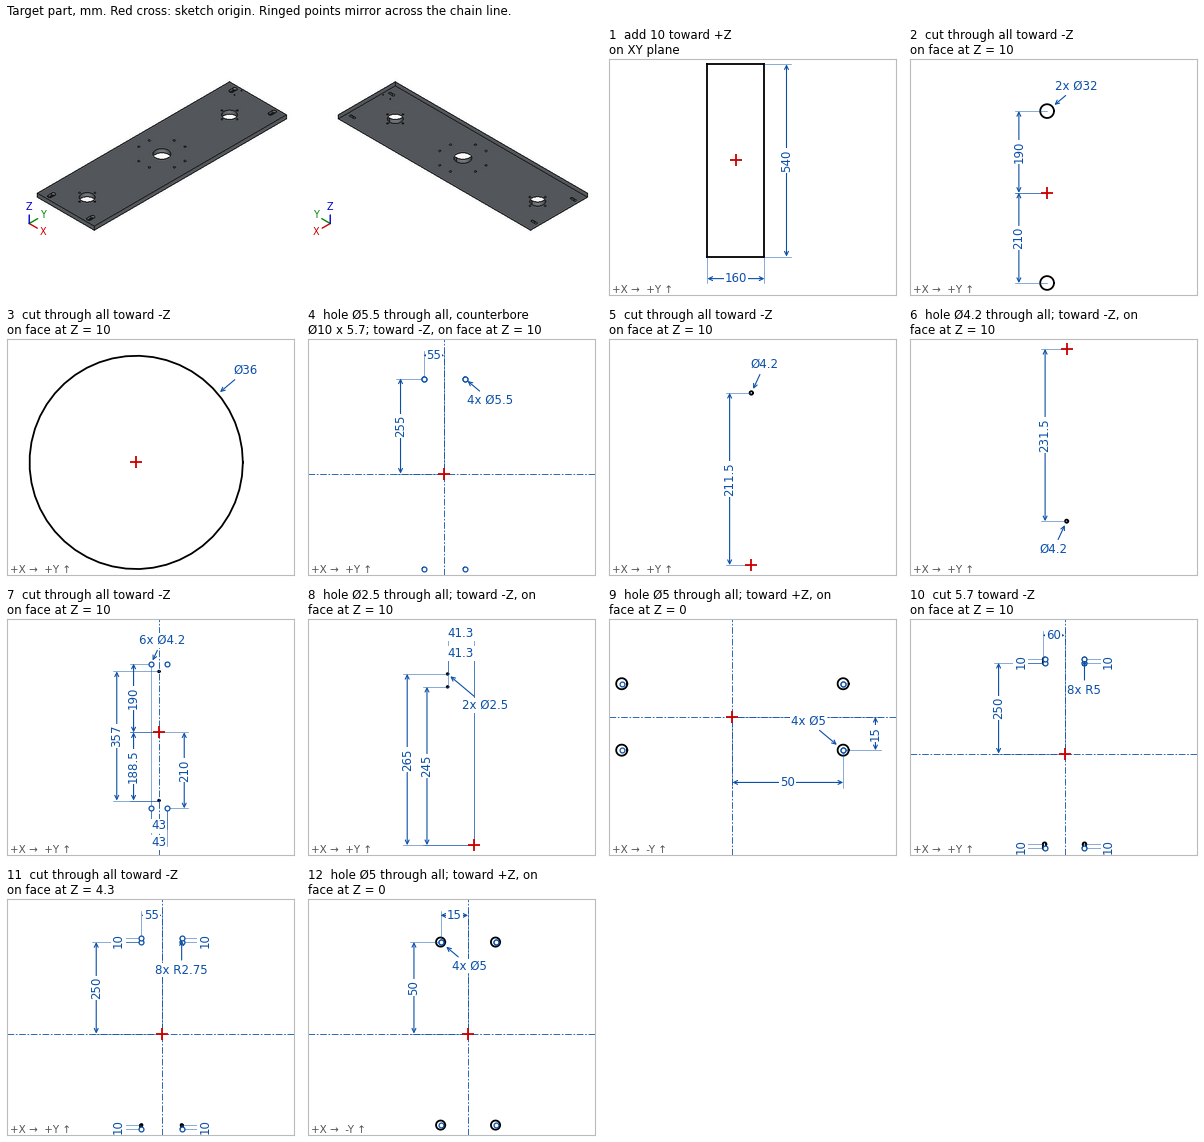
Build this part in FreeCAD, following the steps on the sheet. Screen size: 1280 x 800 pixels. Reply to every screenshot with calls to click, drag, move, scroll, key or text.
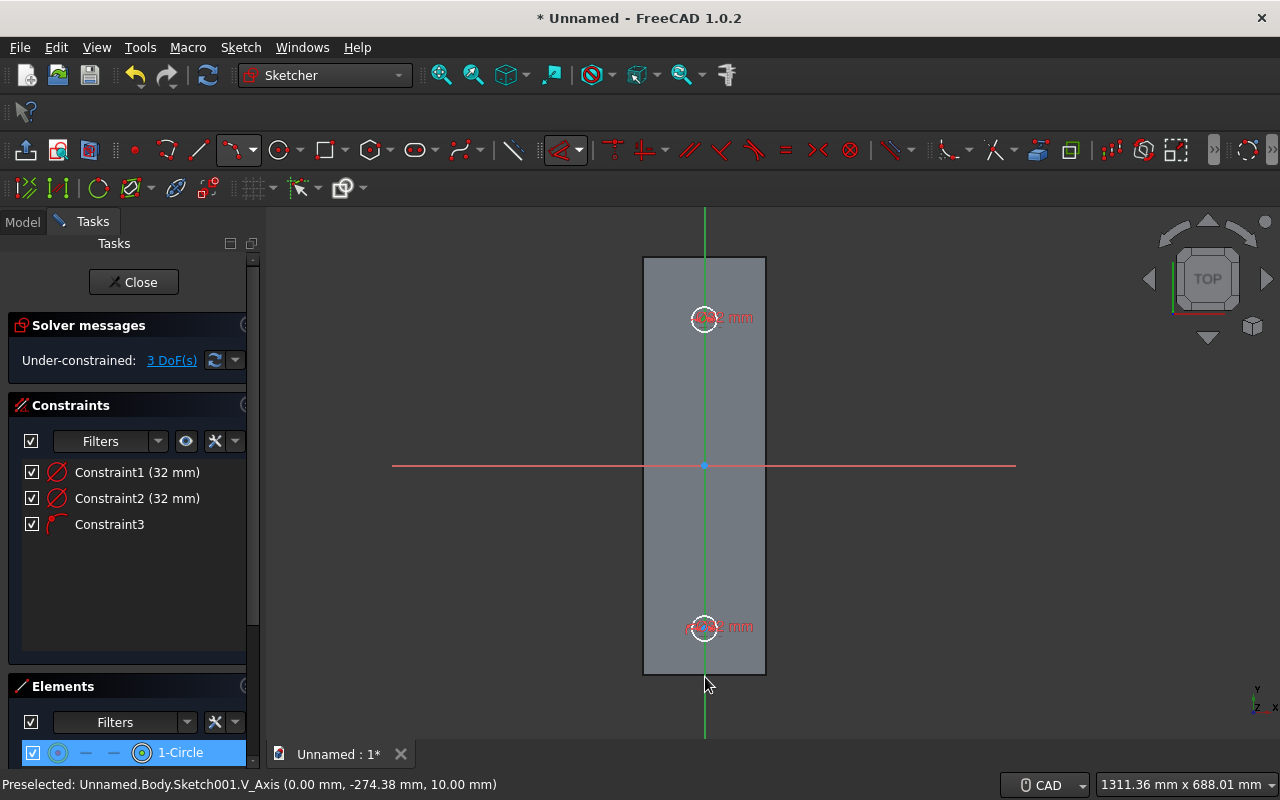
click(614, 150)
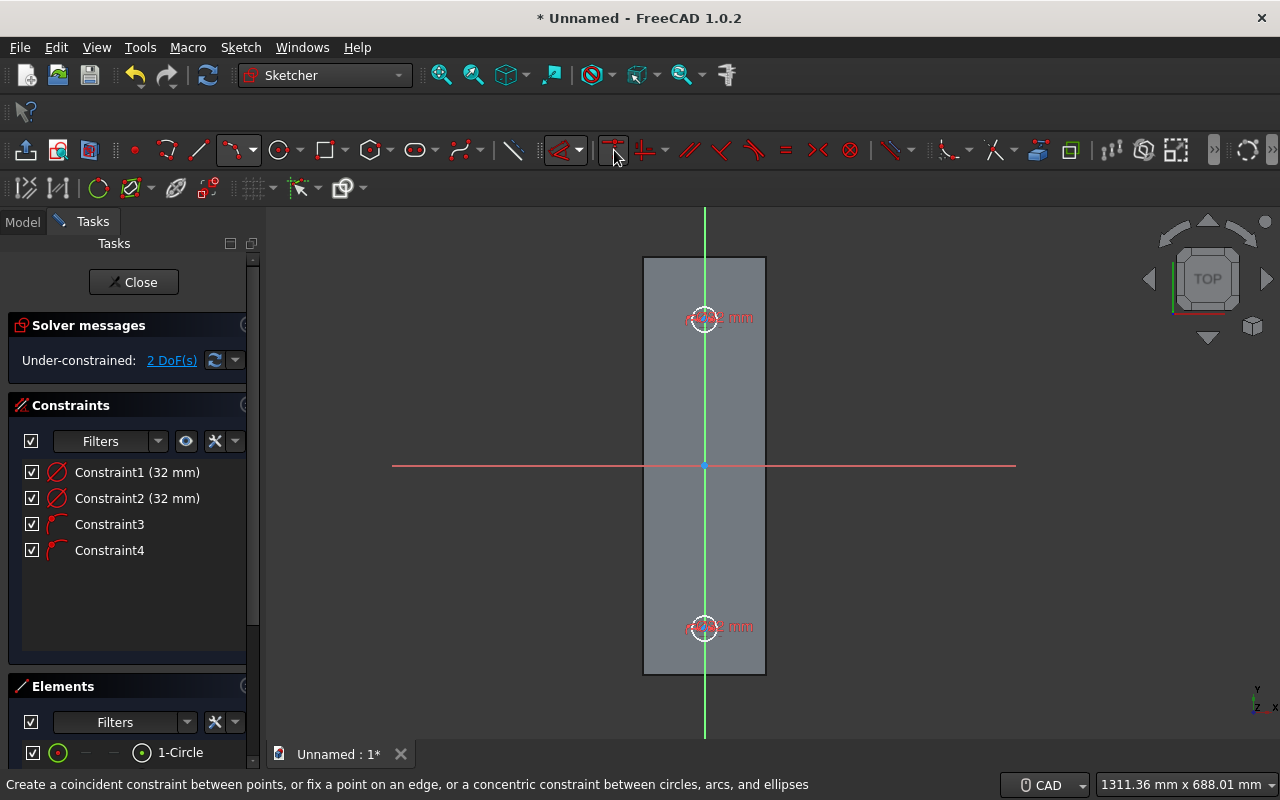
click(560, 150)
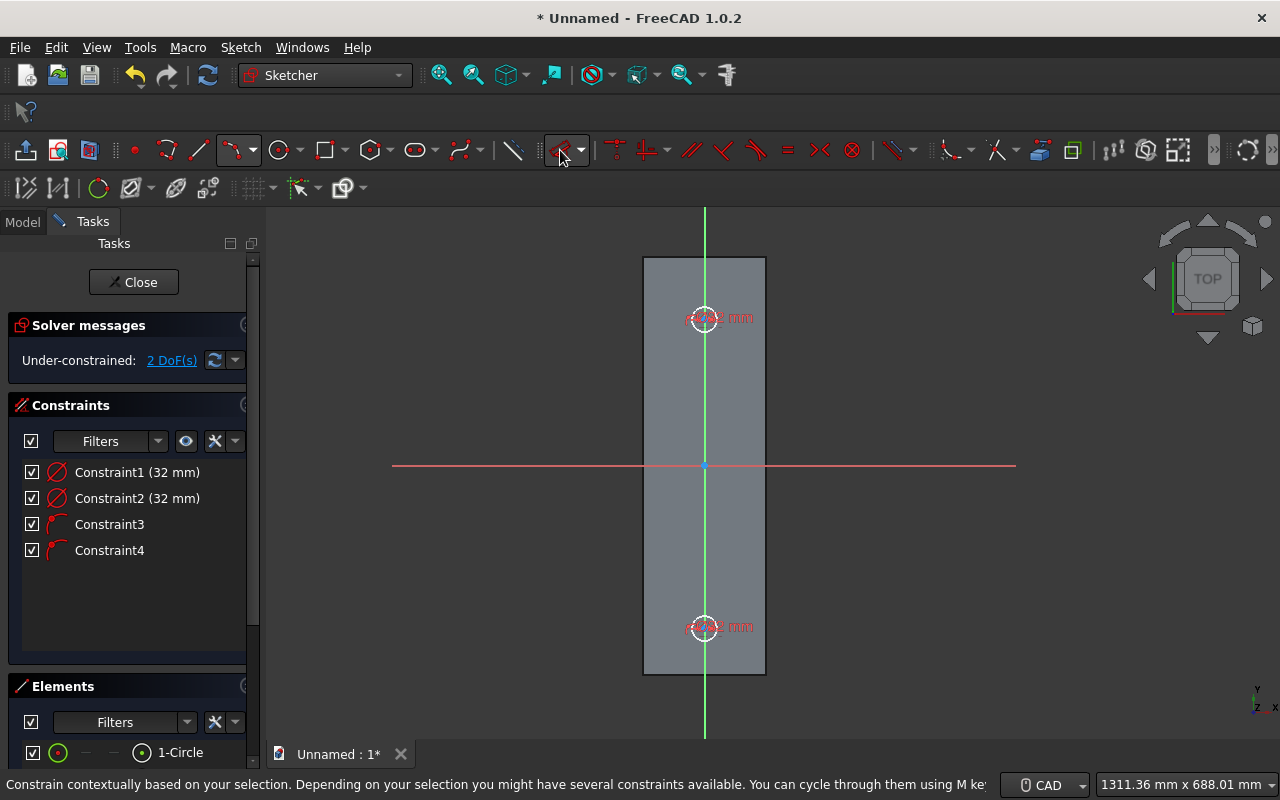
click(705, 320)
click(739, 393)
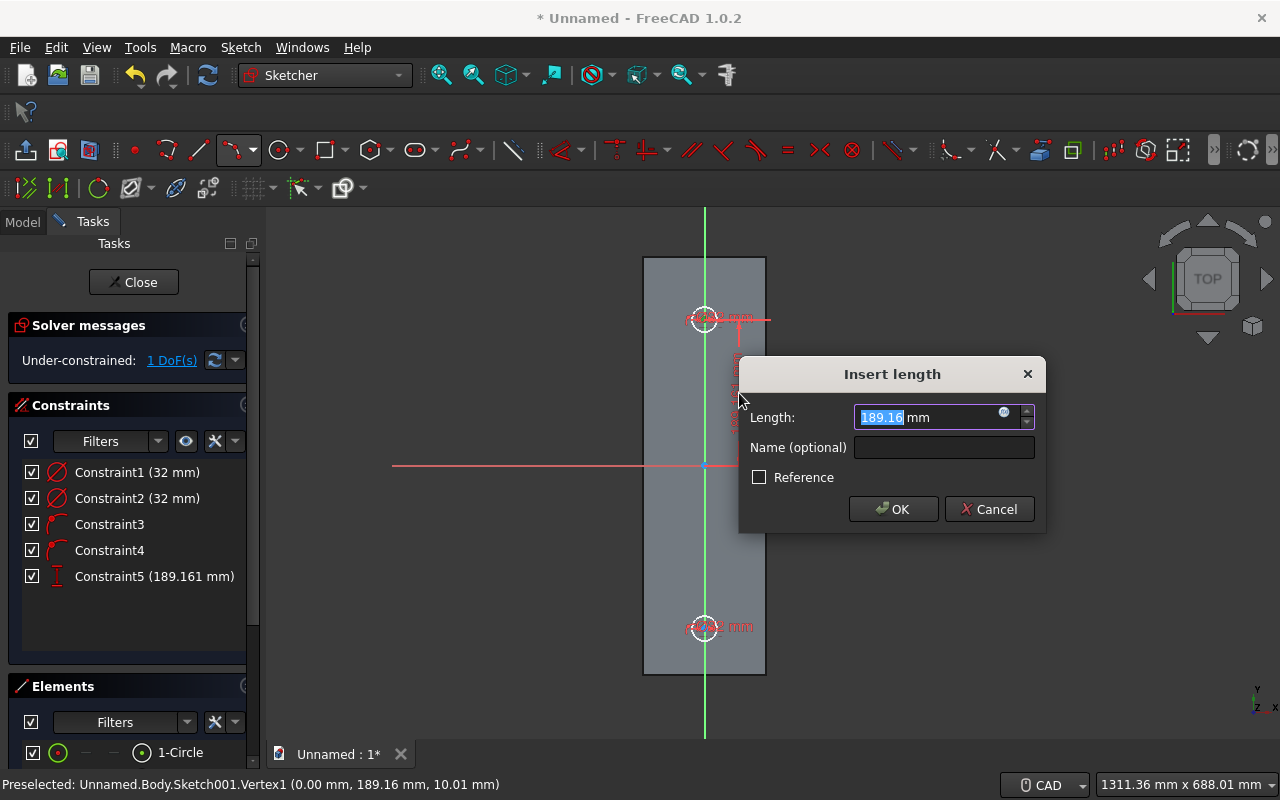
text(190)
key(Return)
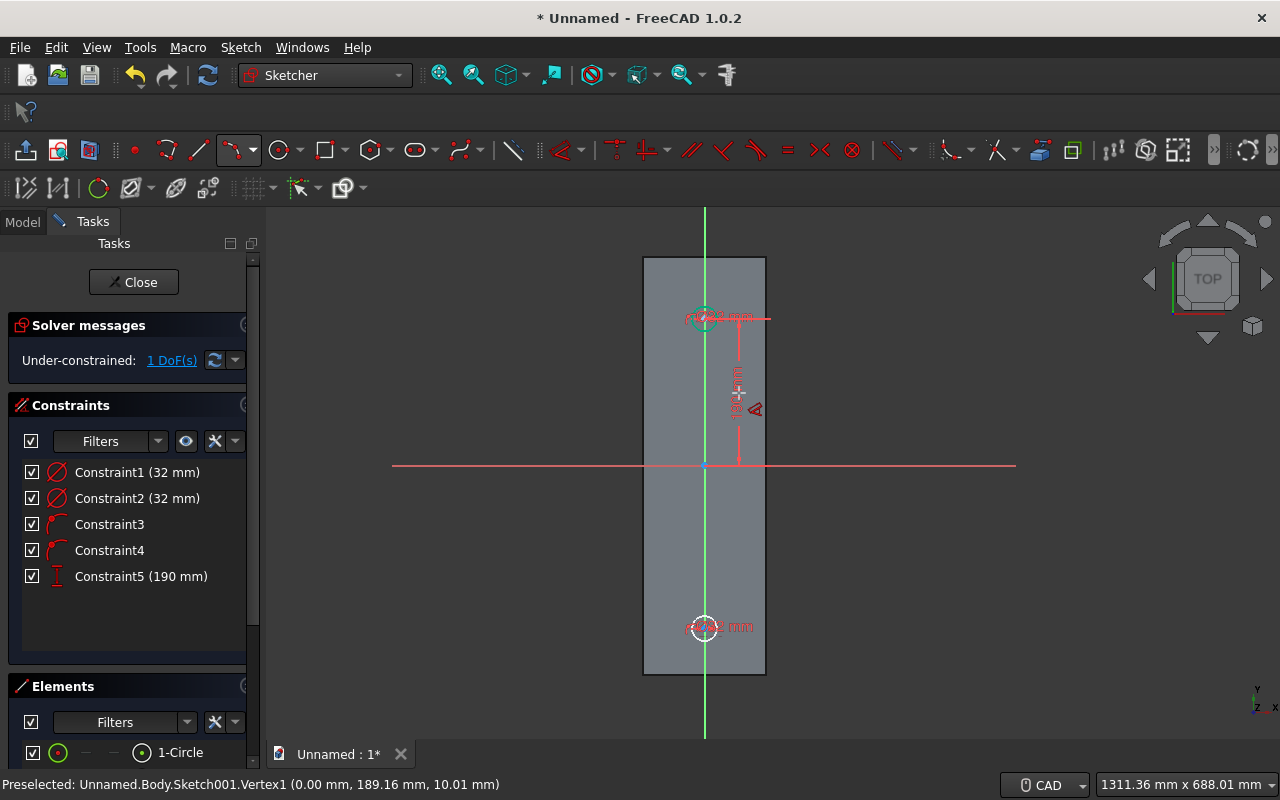
click(705, 629)
click(739, 547)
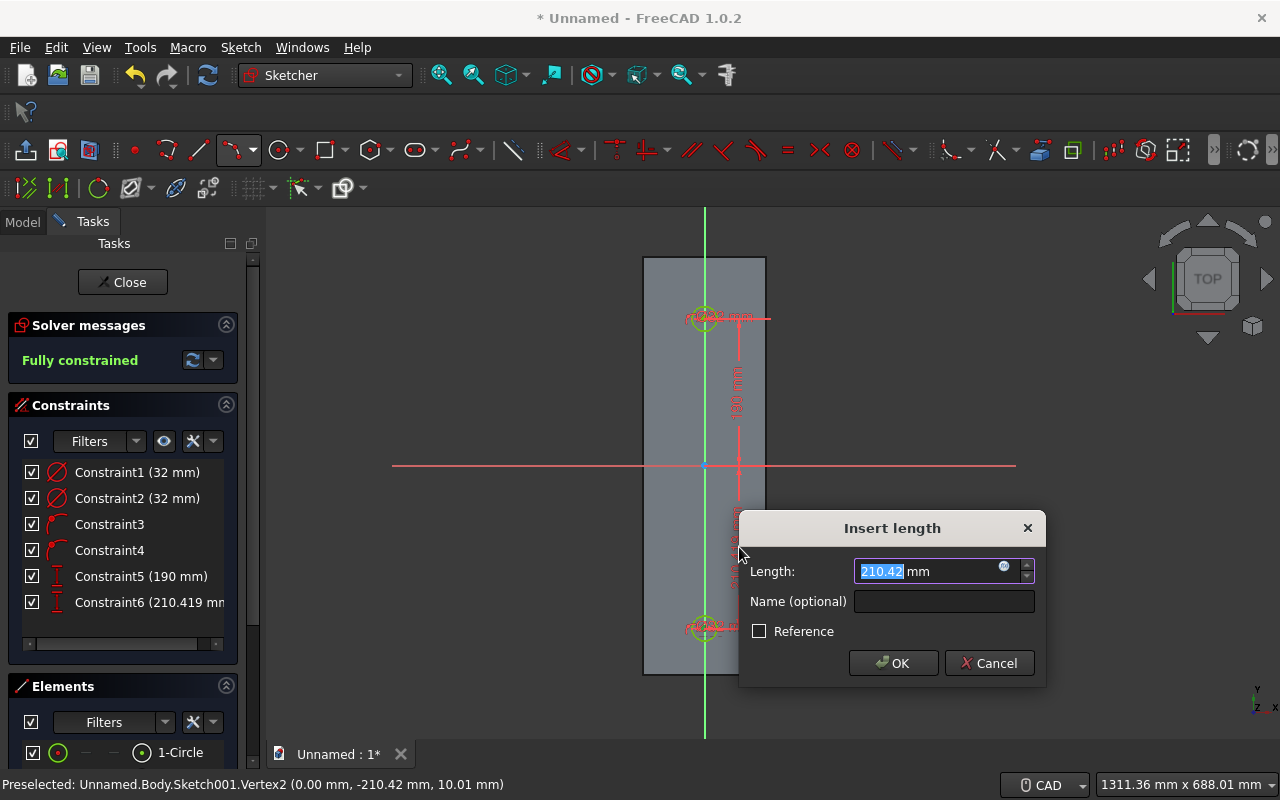
text(210)
key(Return)
key(Escape)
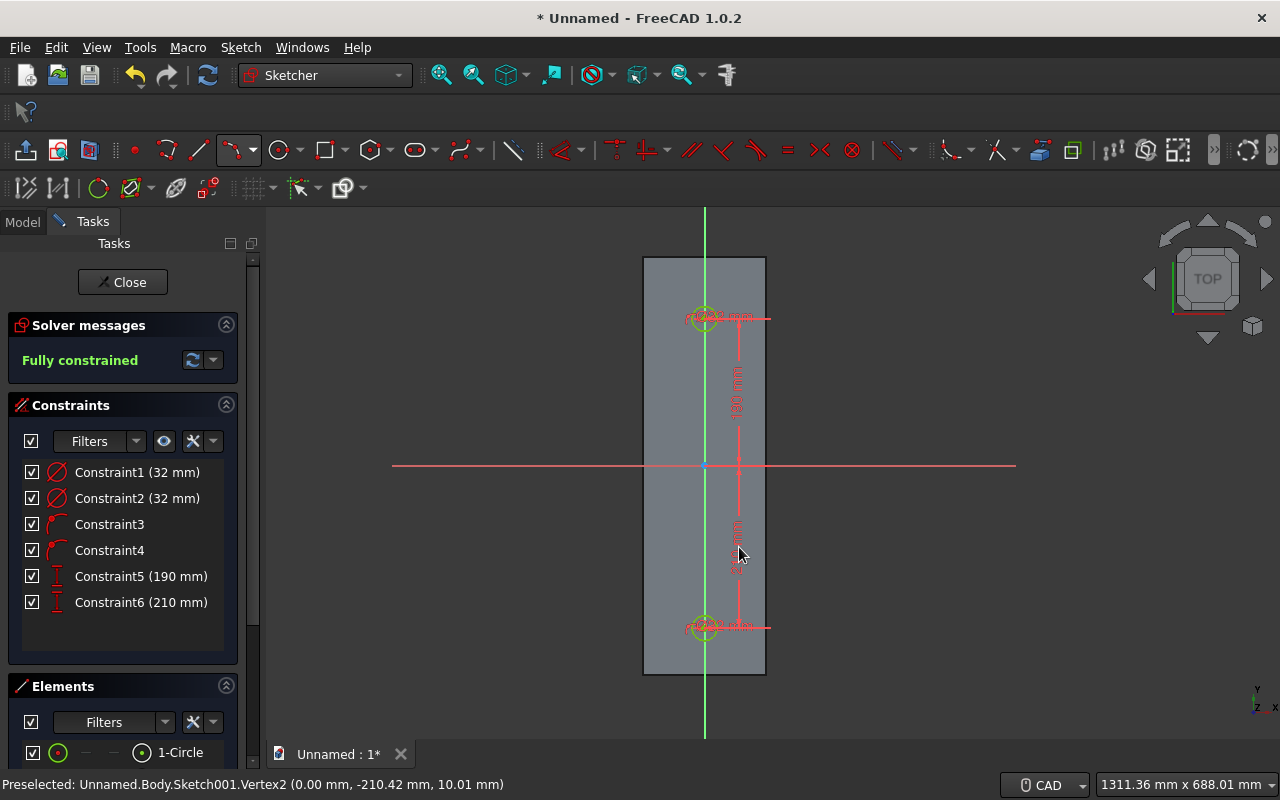
click(123, 282)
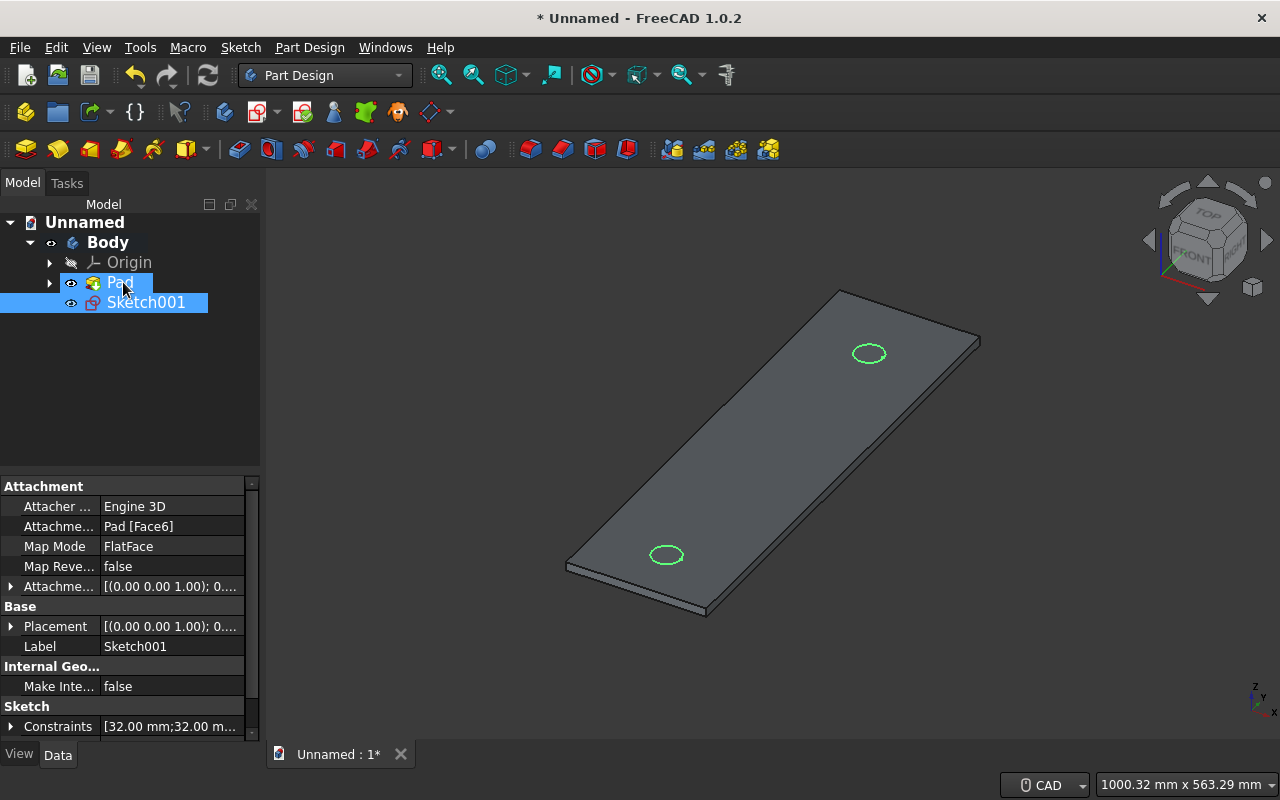
click(240, 150)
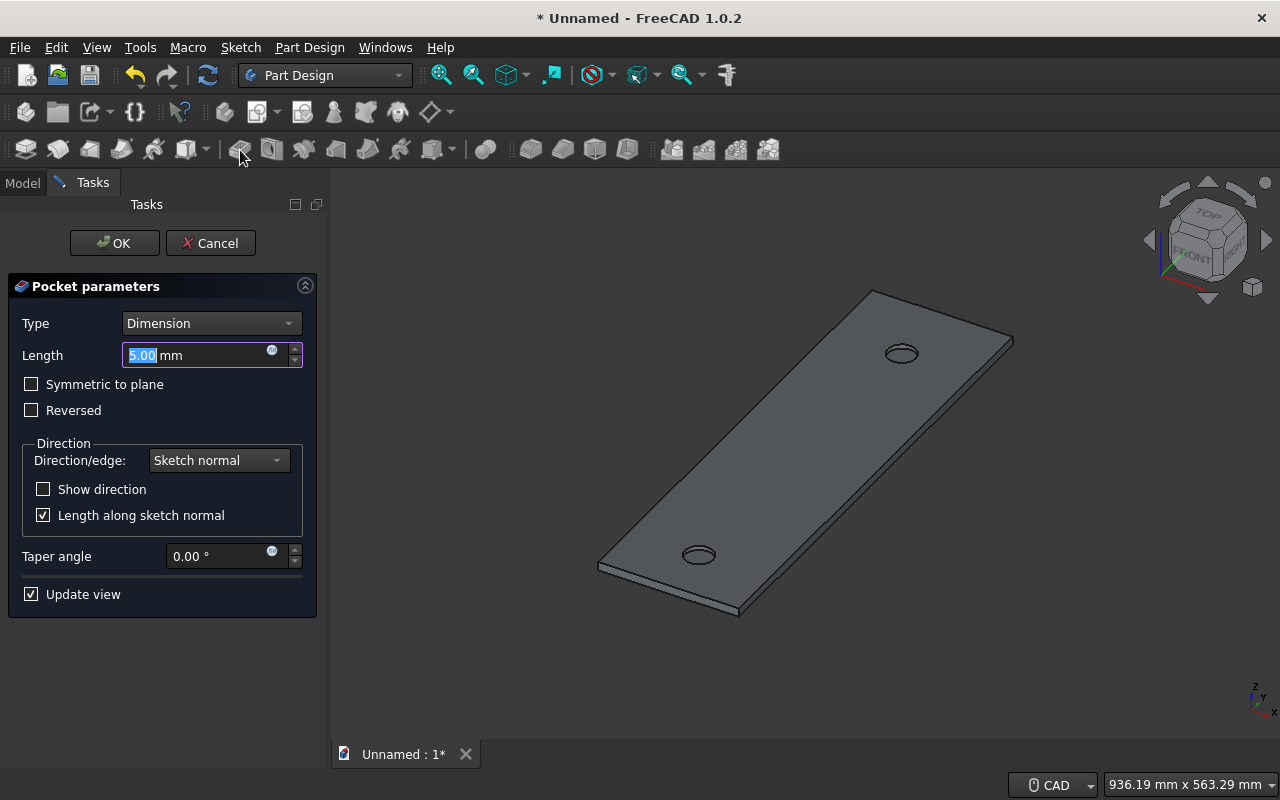
click(212, 324)